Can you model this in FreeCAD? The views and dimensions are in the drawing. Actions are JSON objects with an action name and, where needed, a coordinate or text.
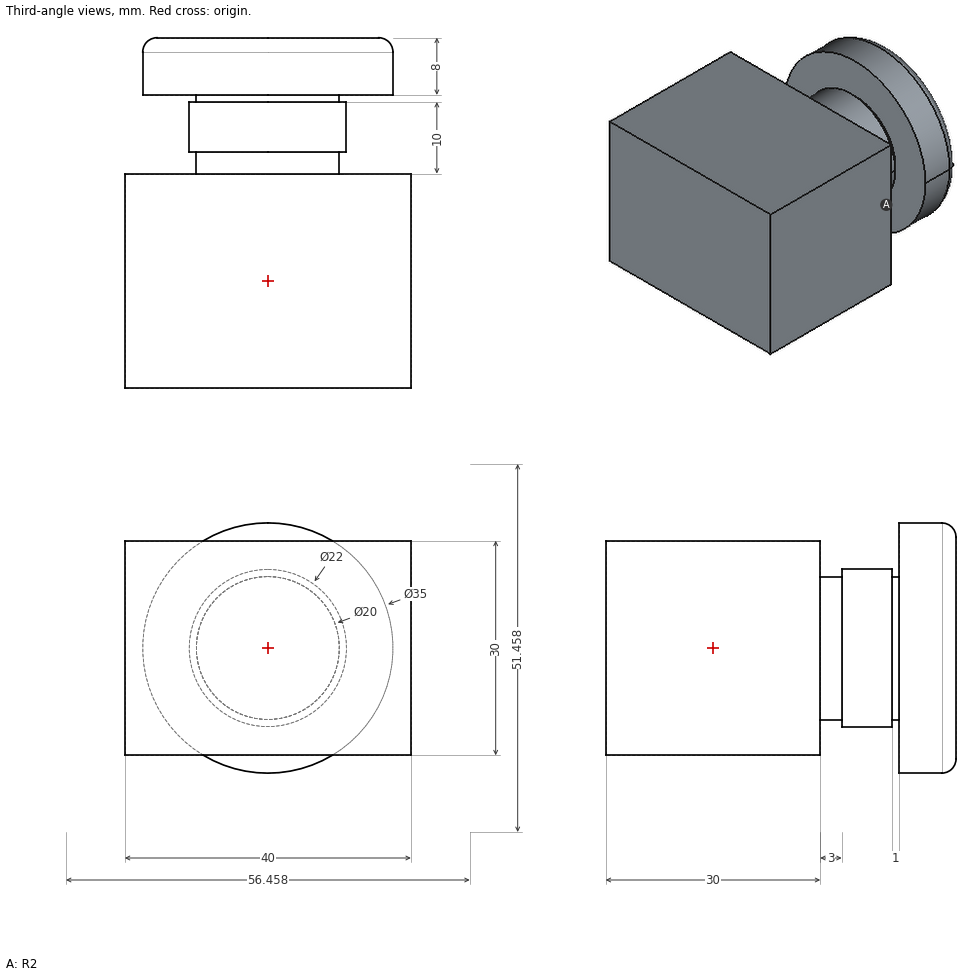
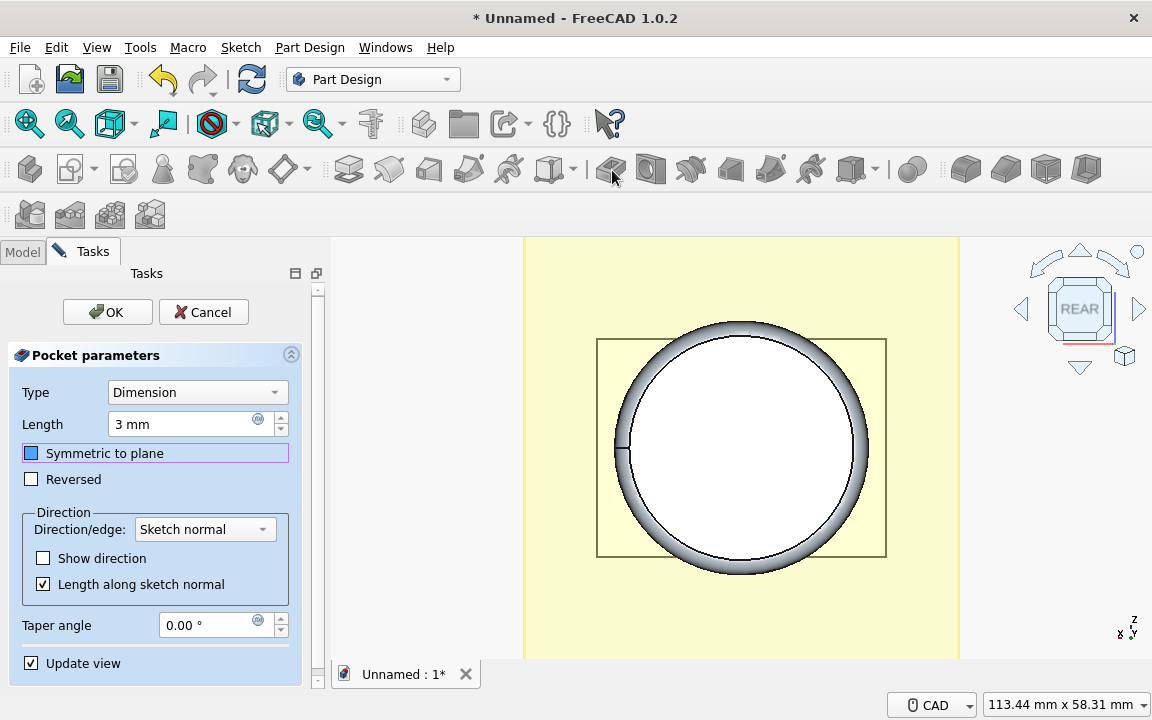
{"action": "left_click", "coordinate": [30, 479]}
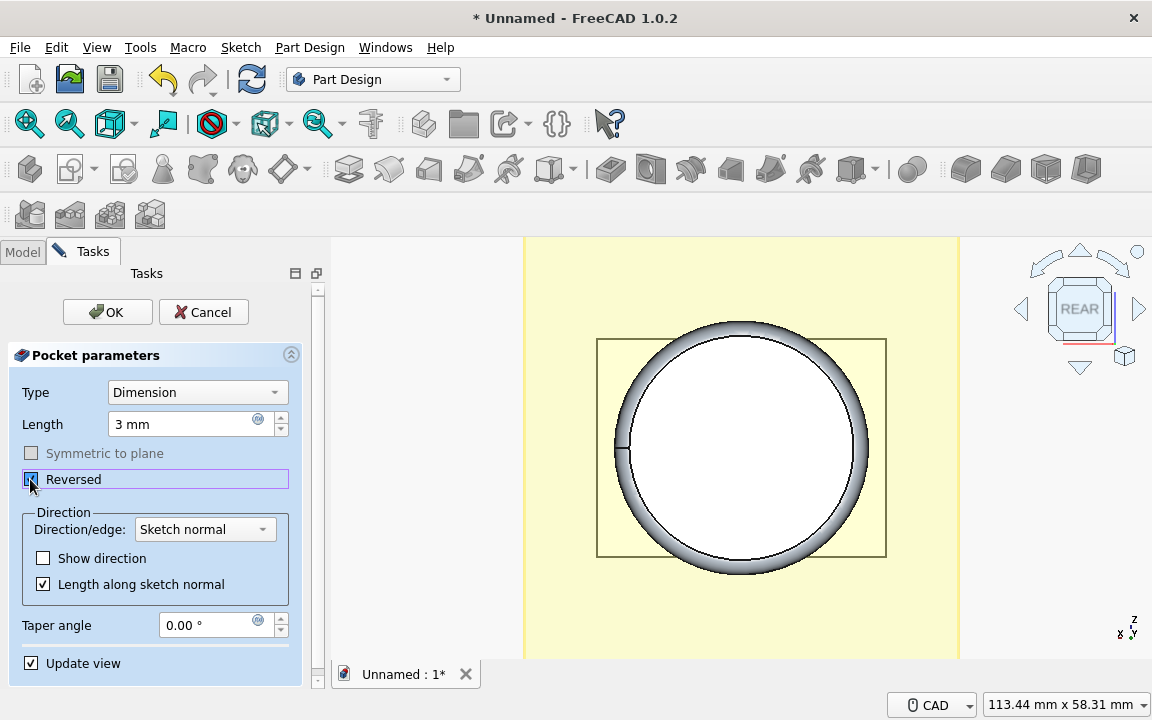
{"action": "left_click", "coordinate": [108, 312]}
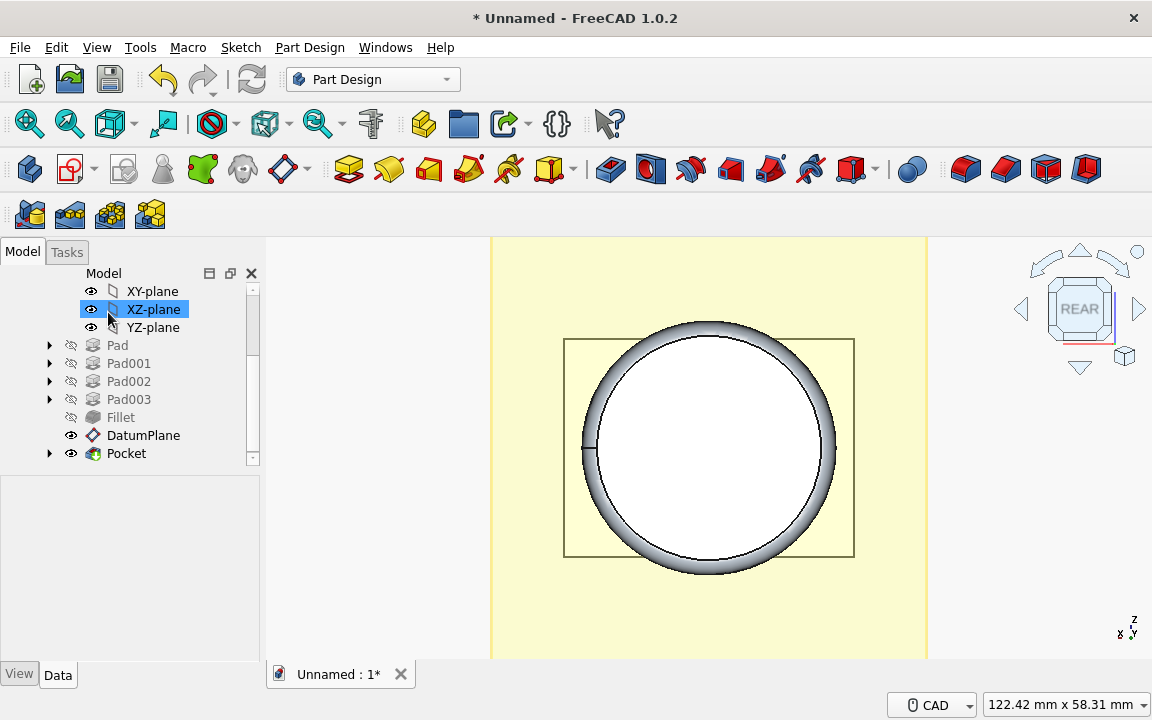
{"action": "left_click", "coordinate": [116, 435]}
{"action": "key", "text": "space"}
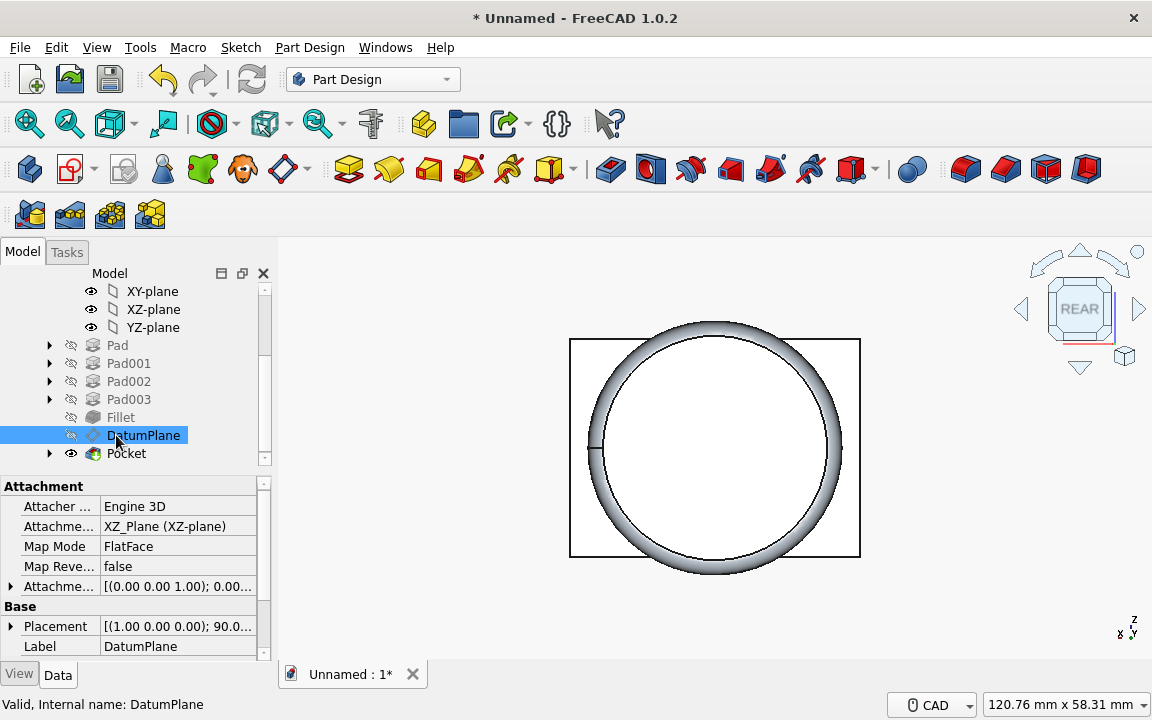
{"action": "key", "text": "0"}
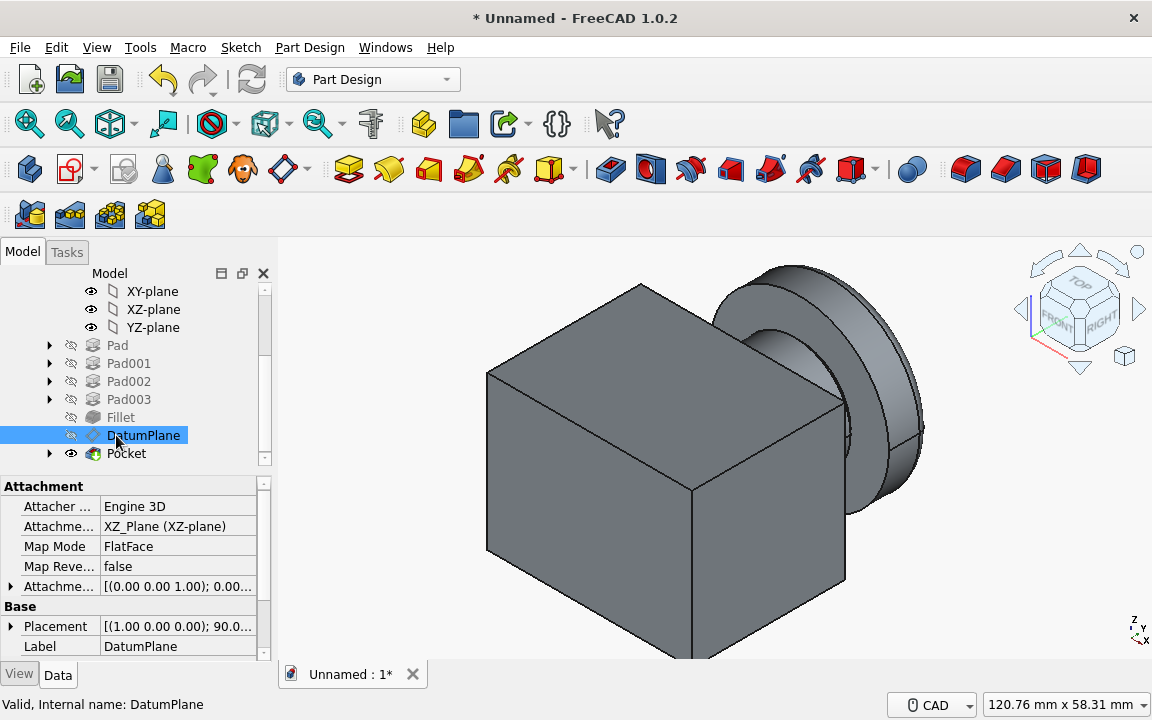
{"action": "left_click", "coordinate": [30, 124]}